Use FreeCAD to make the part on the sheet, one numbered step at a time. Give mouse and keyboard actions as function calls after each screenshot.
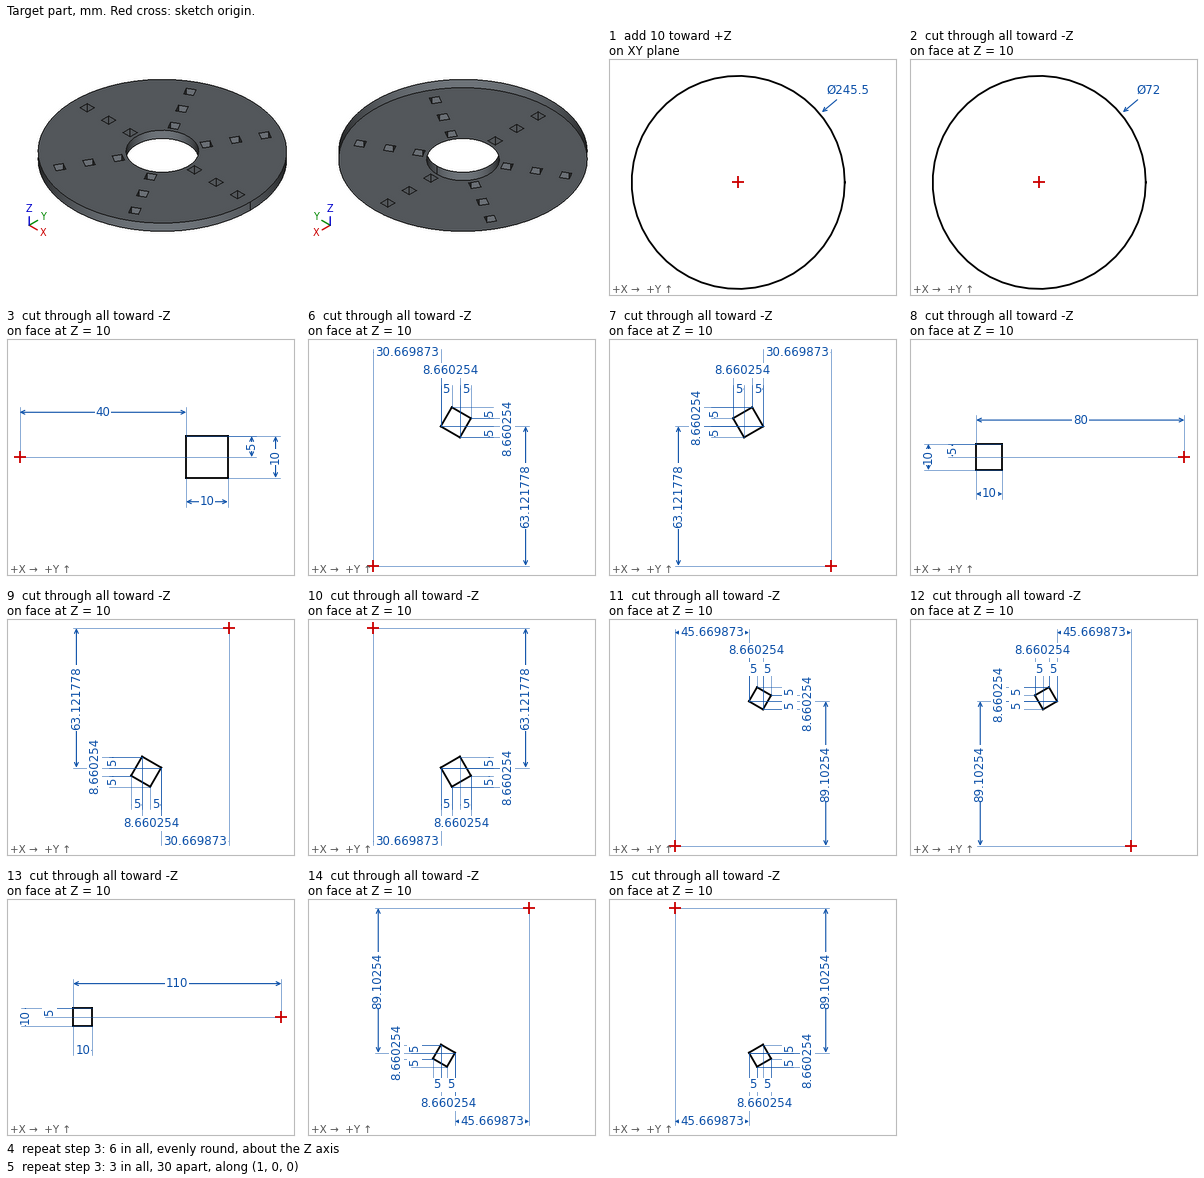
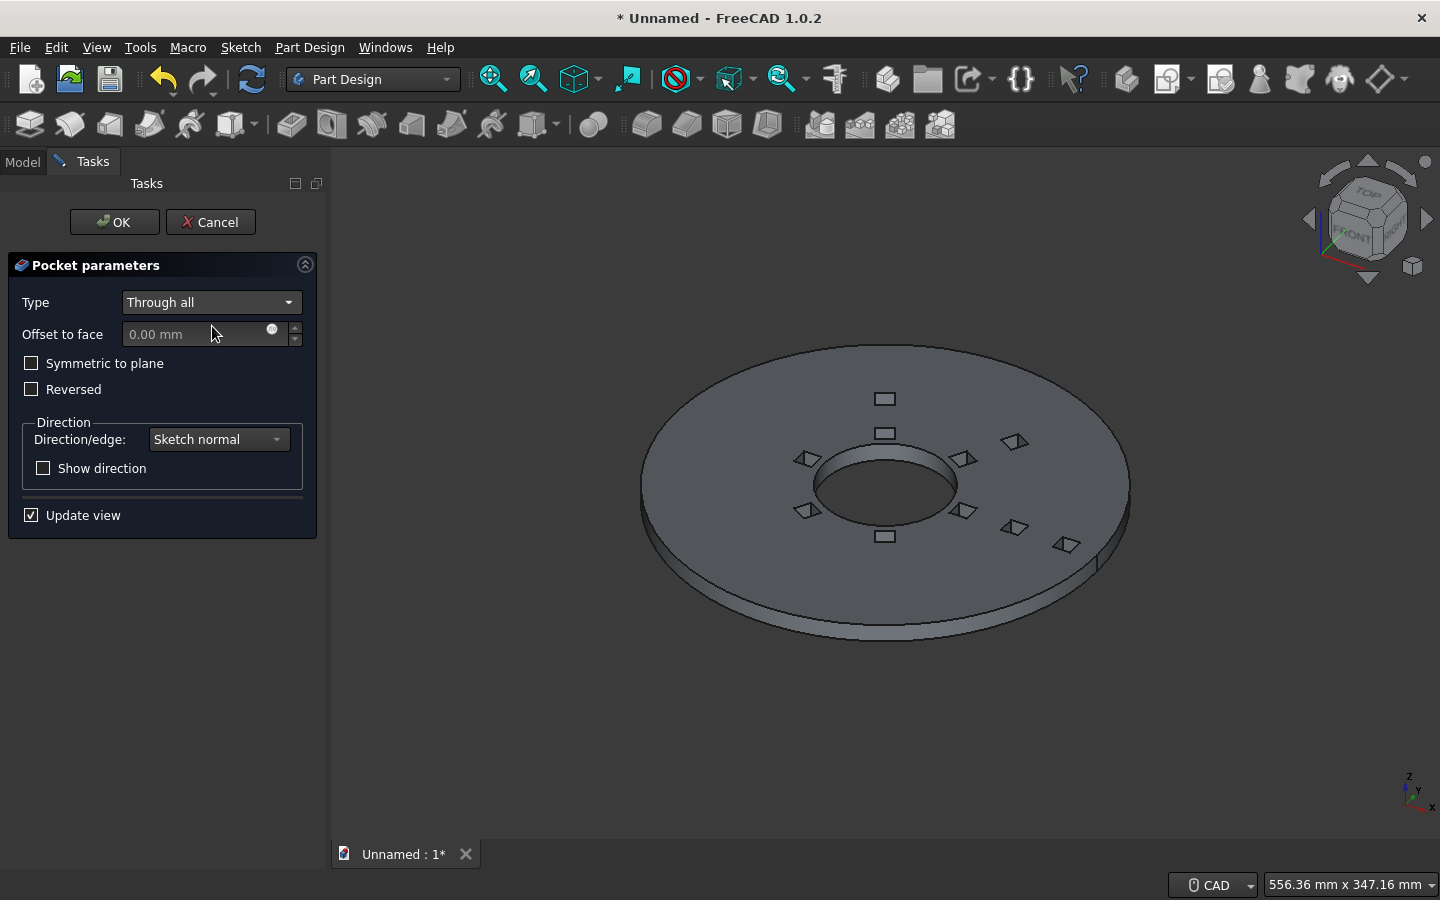
click(115, 222)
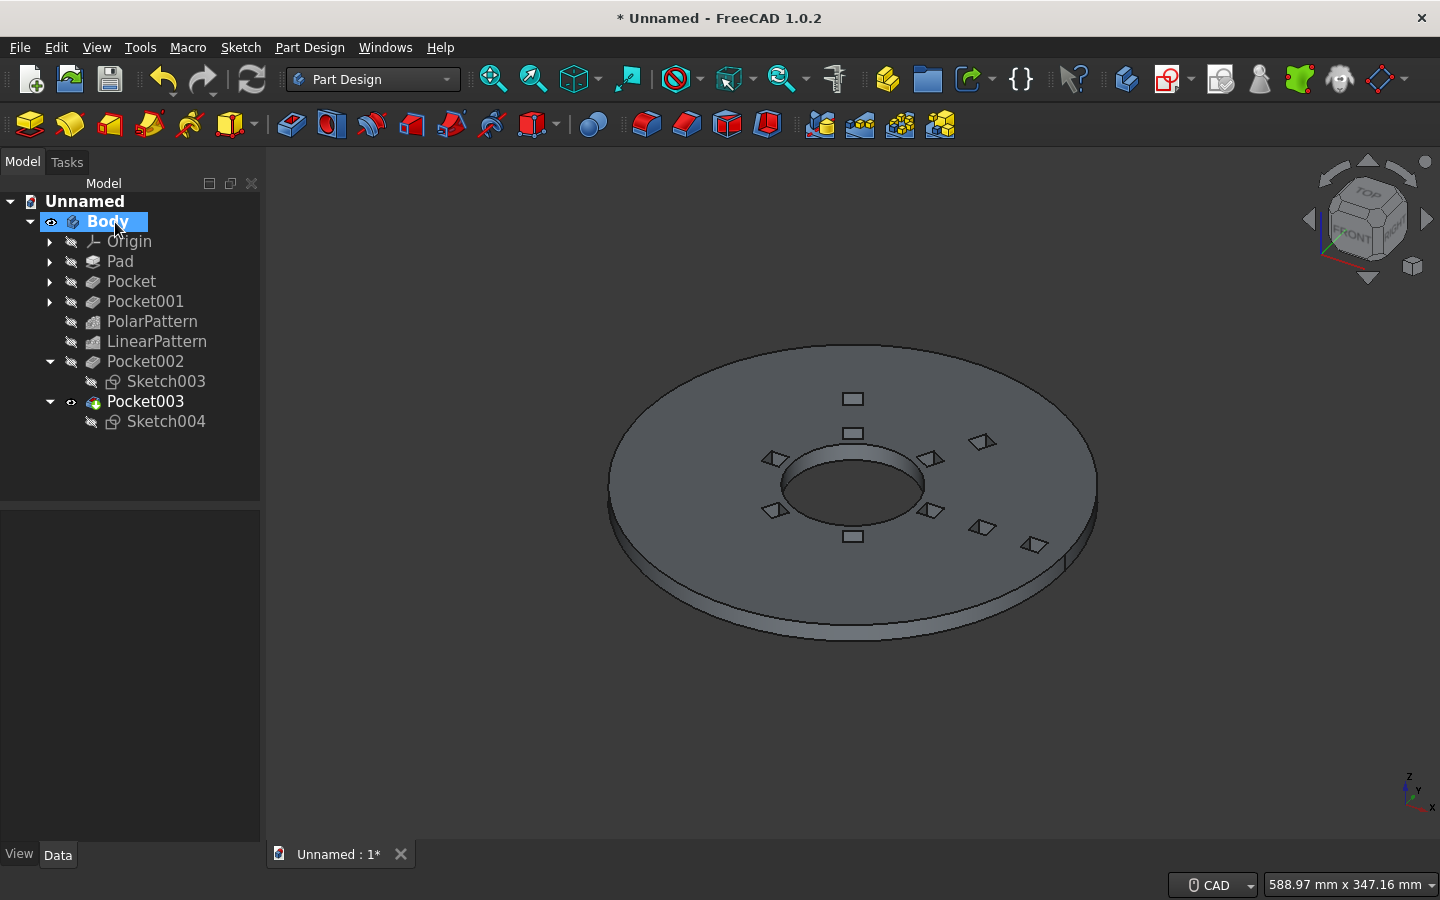
click(767, 409)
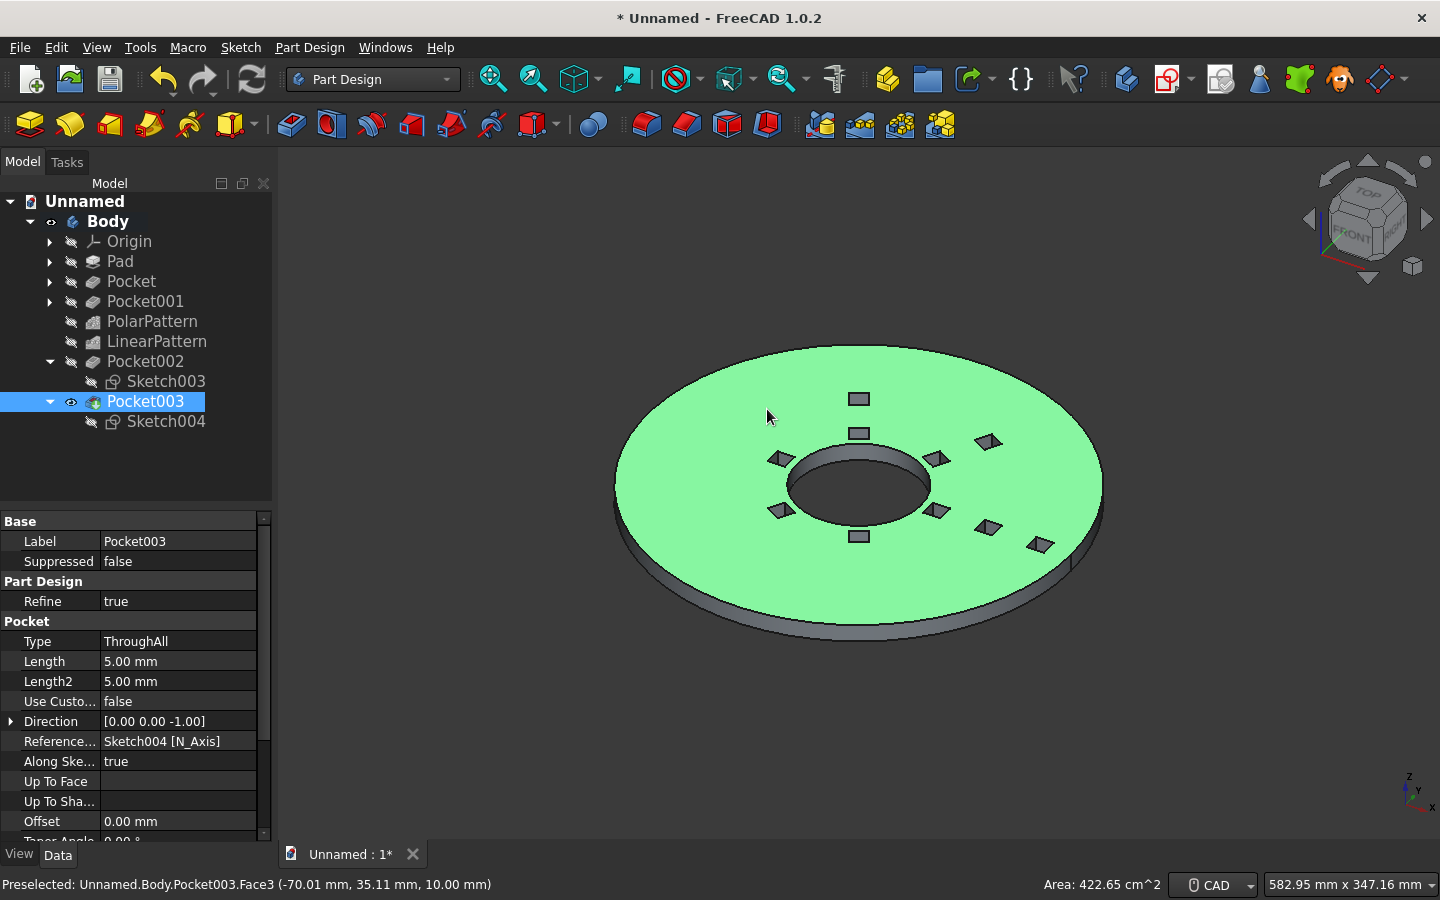
click(1168, 80)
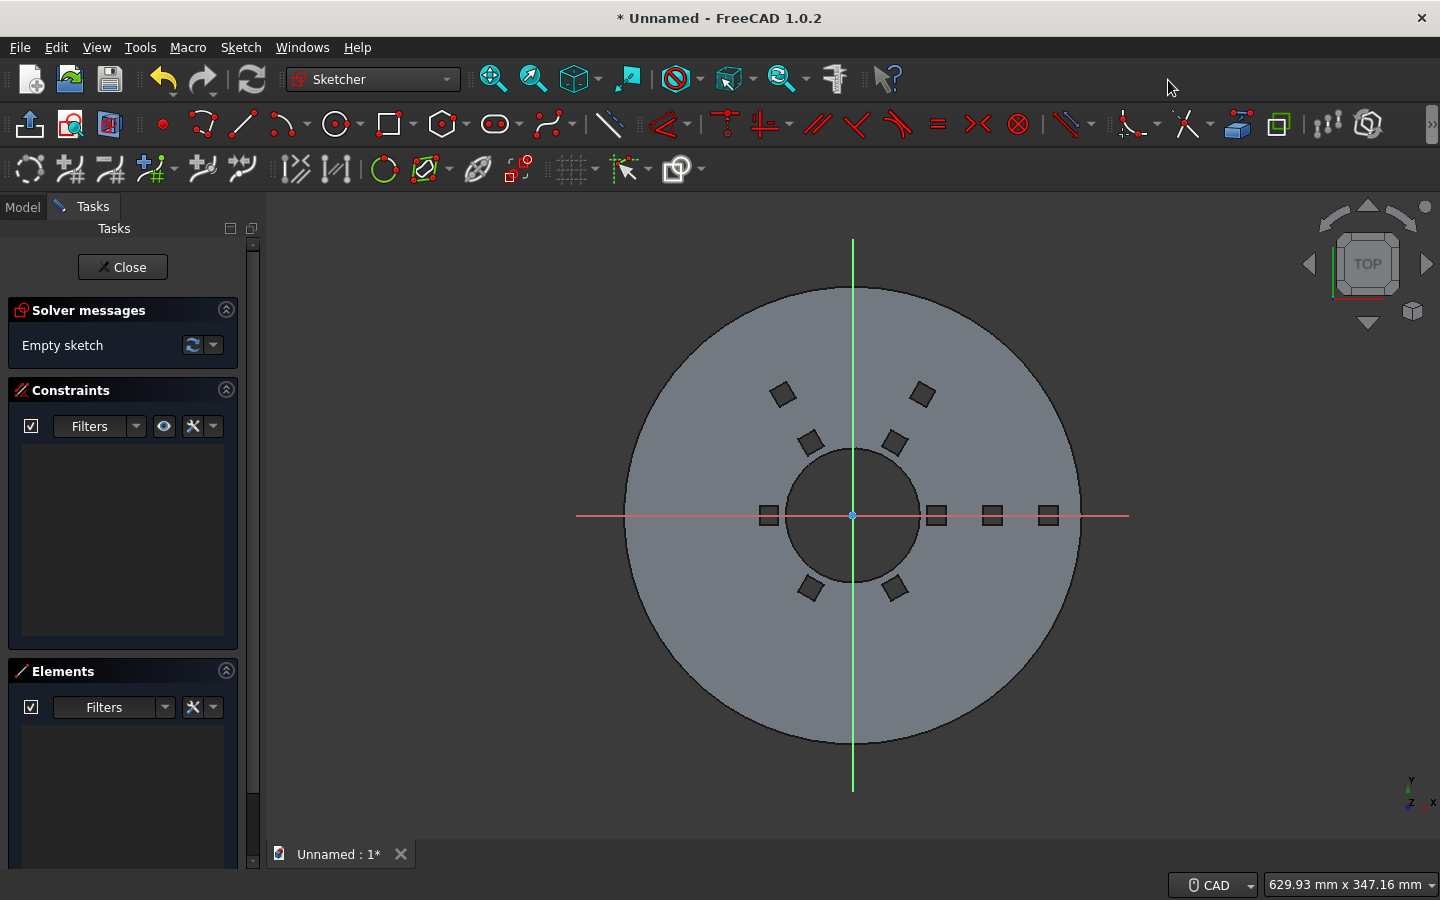
scroll(709, 516, up, 15)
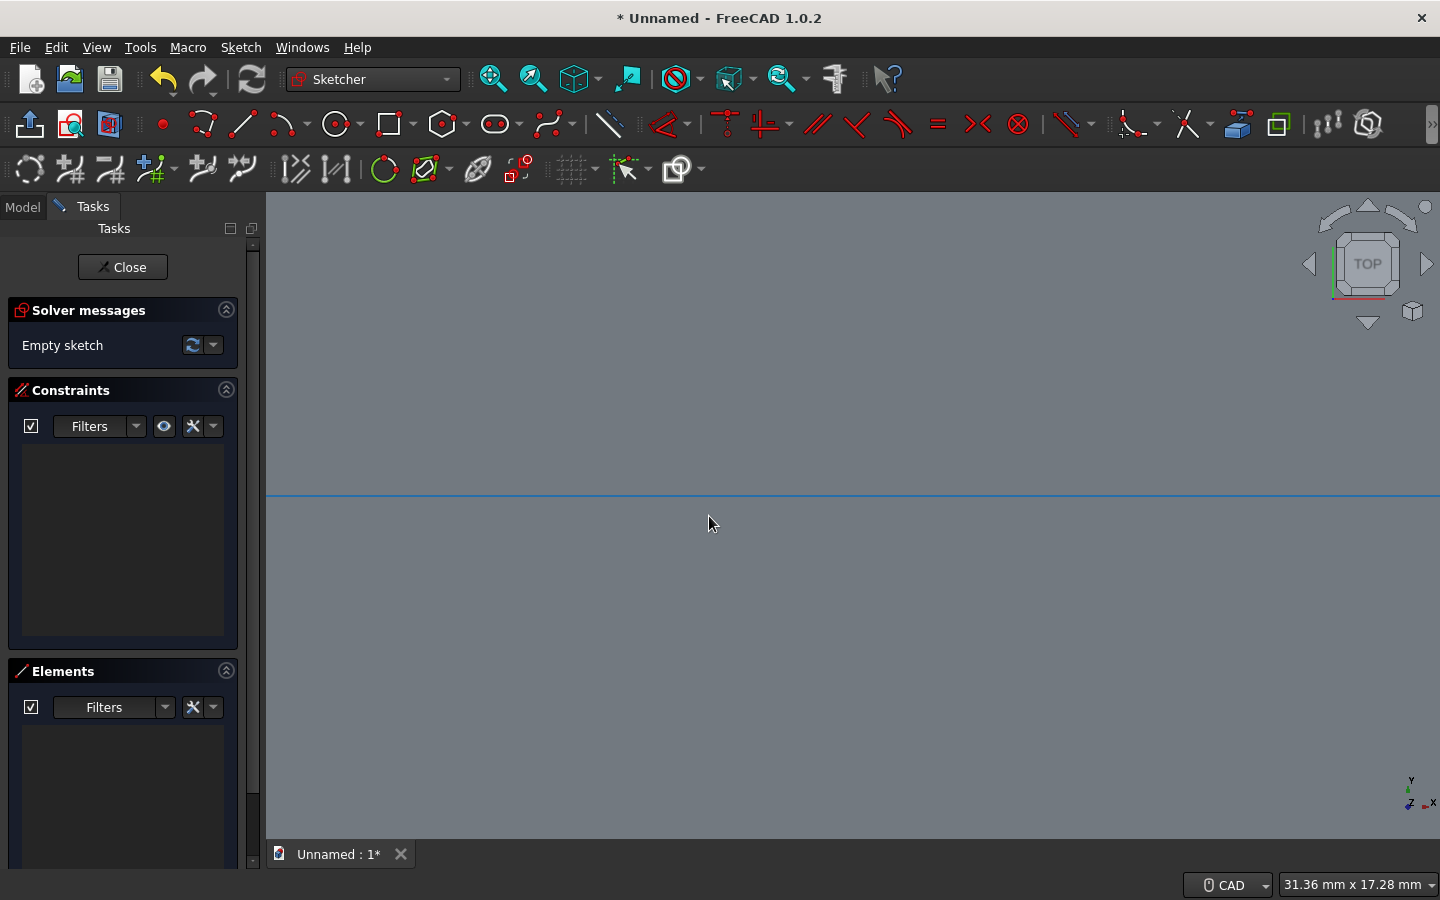
key(g)
key(r)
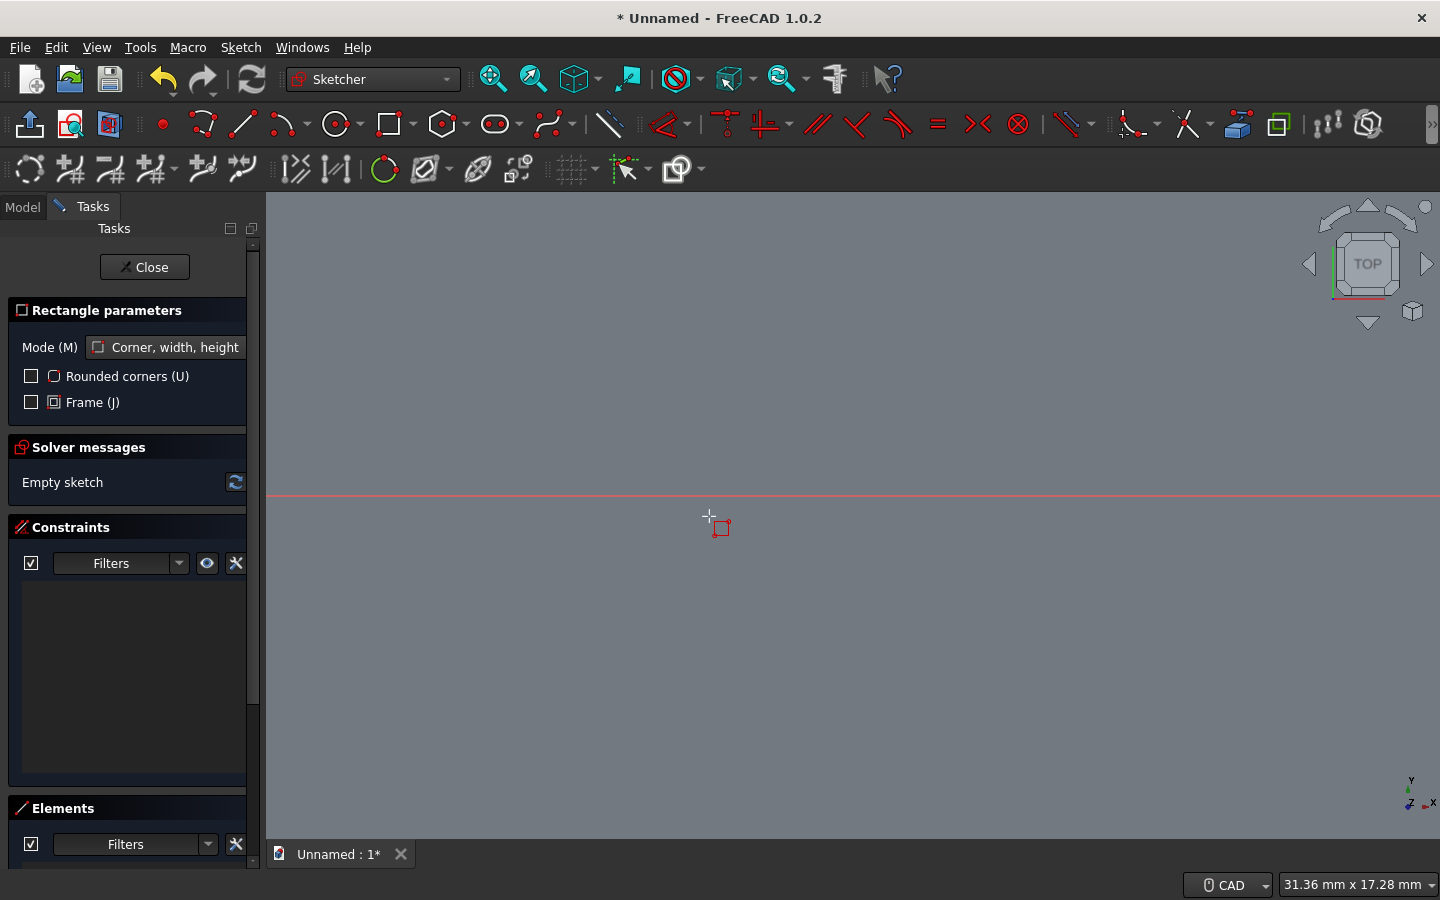
click(596, 309)
move(971, 684)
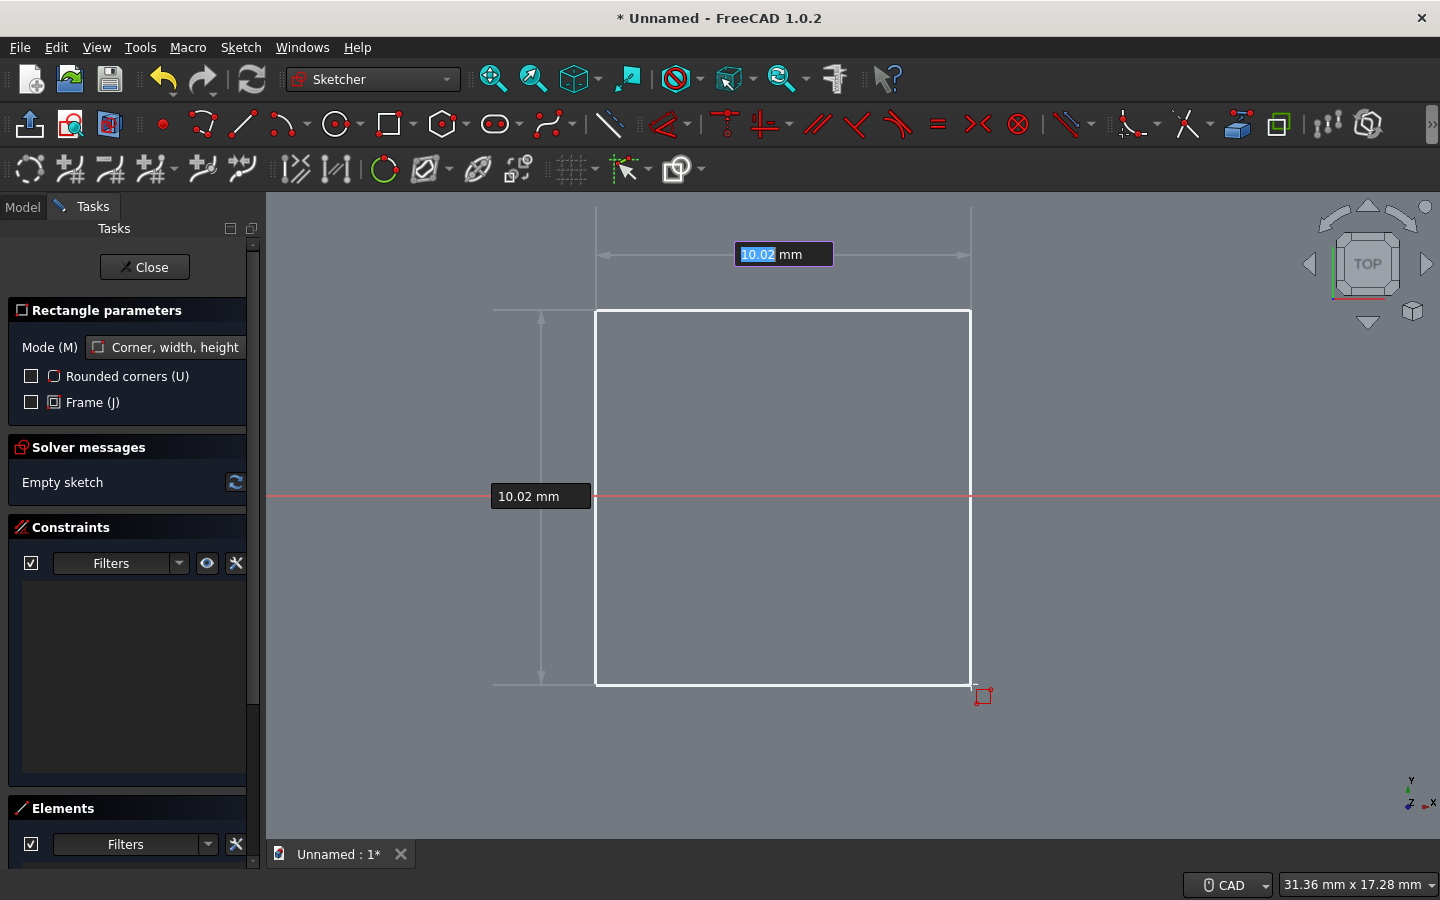
text(10)
key(Tab)
text(10)
key(Return)
key(Escape)